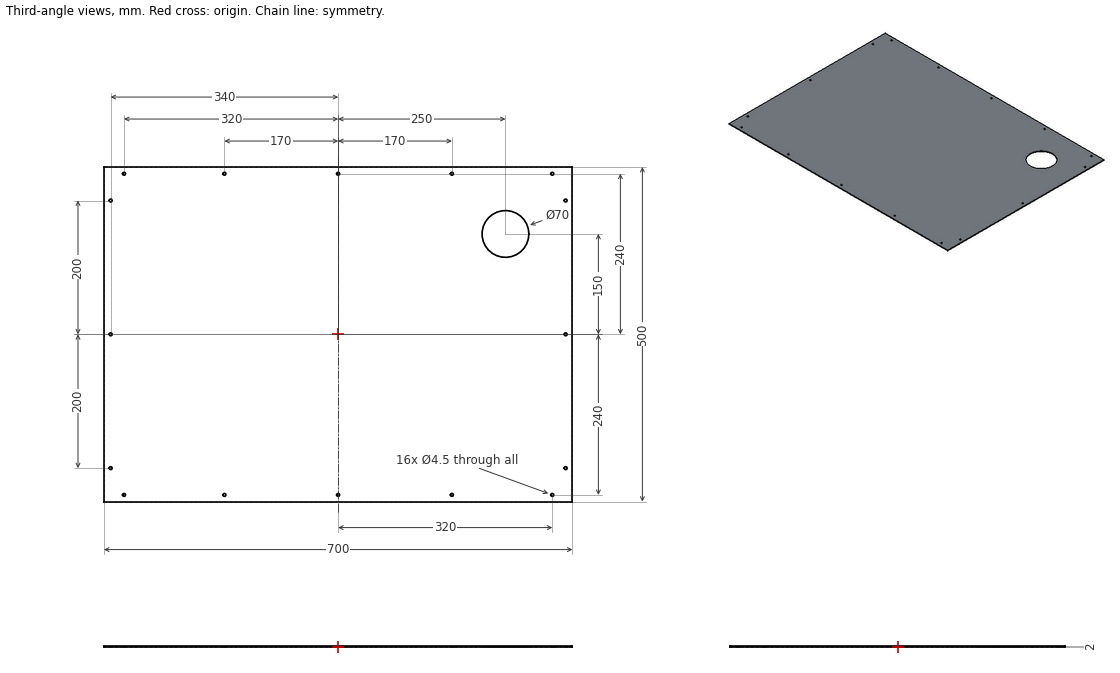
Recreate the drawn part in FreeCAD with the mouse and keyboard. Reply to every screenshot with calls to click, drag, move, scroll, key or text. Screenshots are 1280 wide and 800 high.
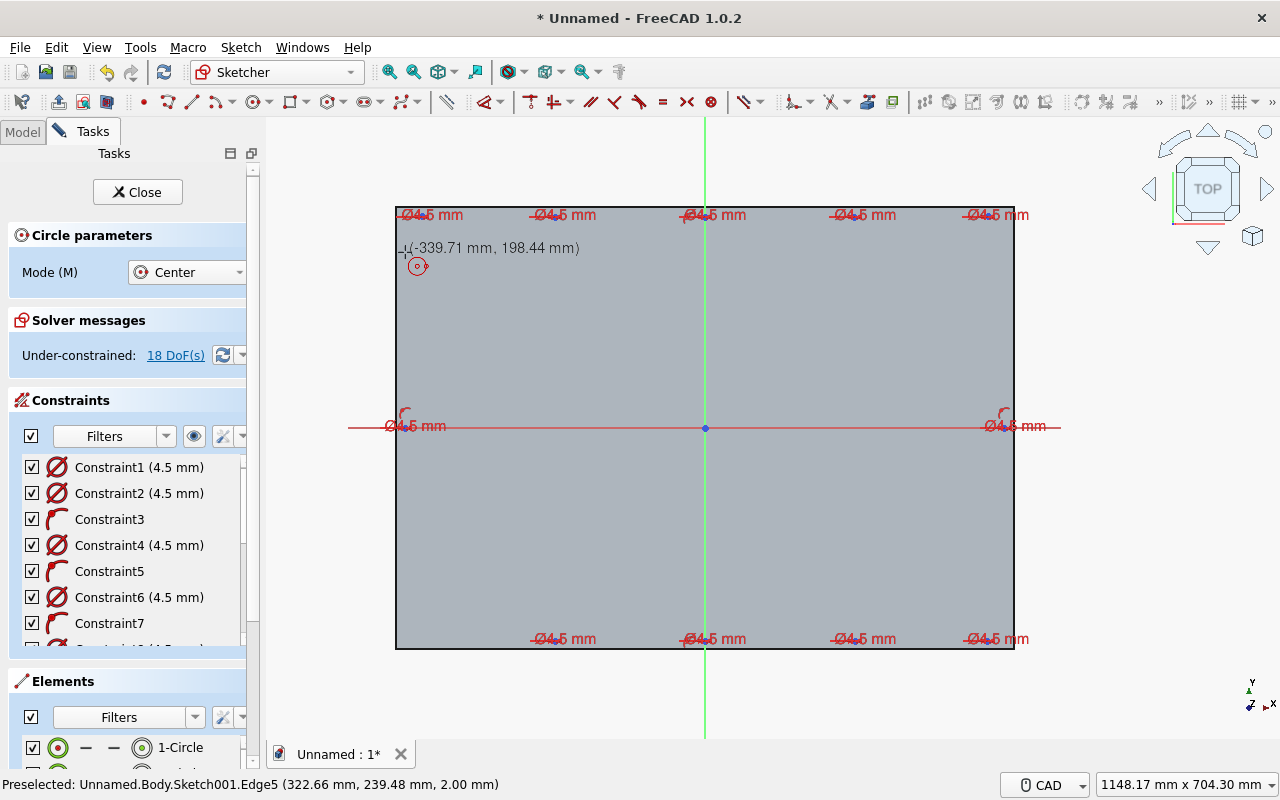
click(405, 252)
move(406, 250)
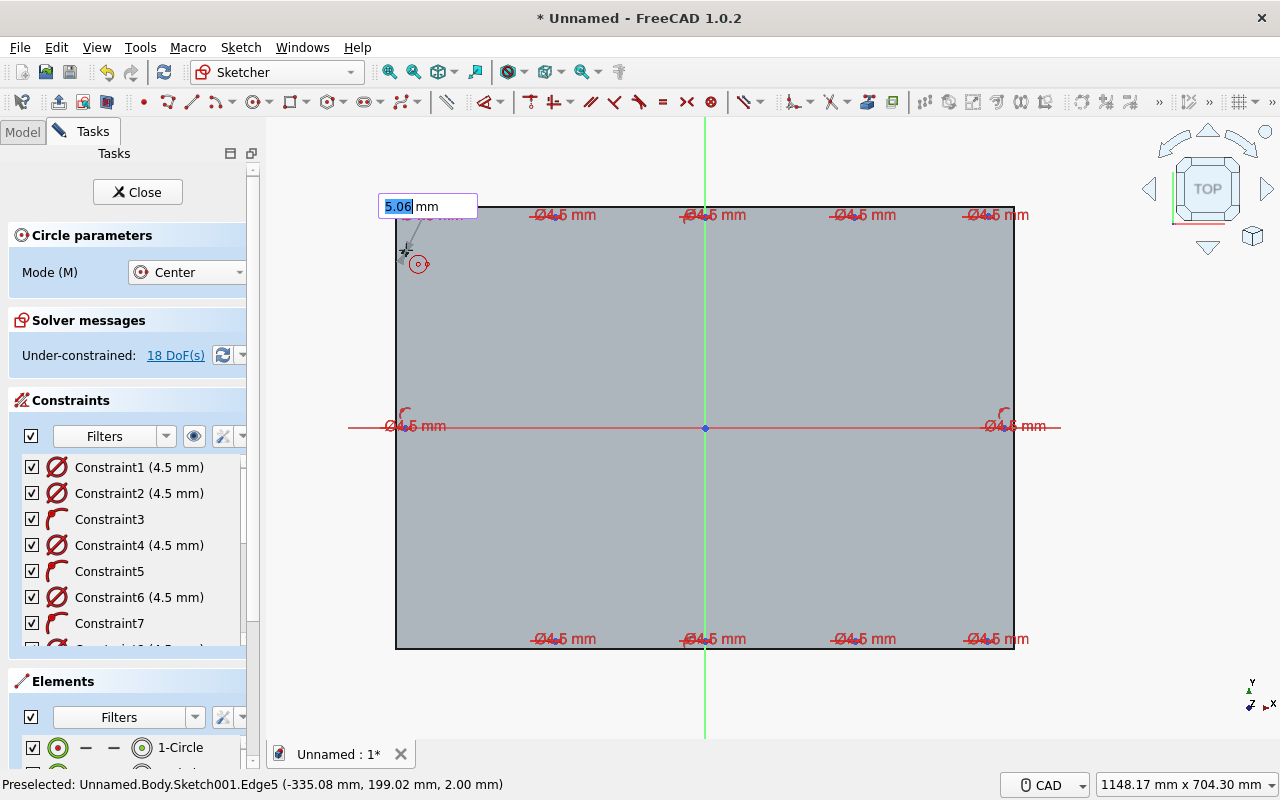
text(4.5)
key(Return)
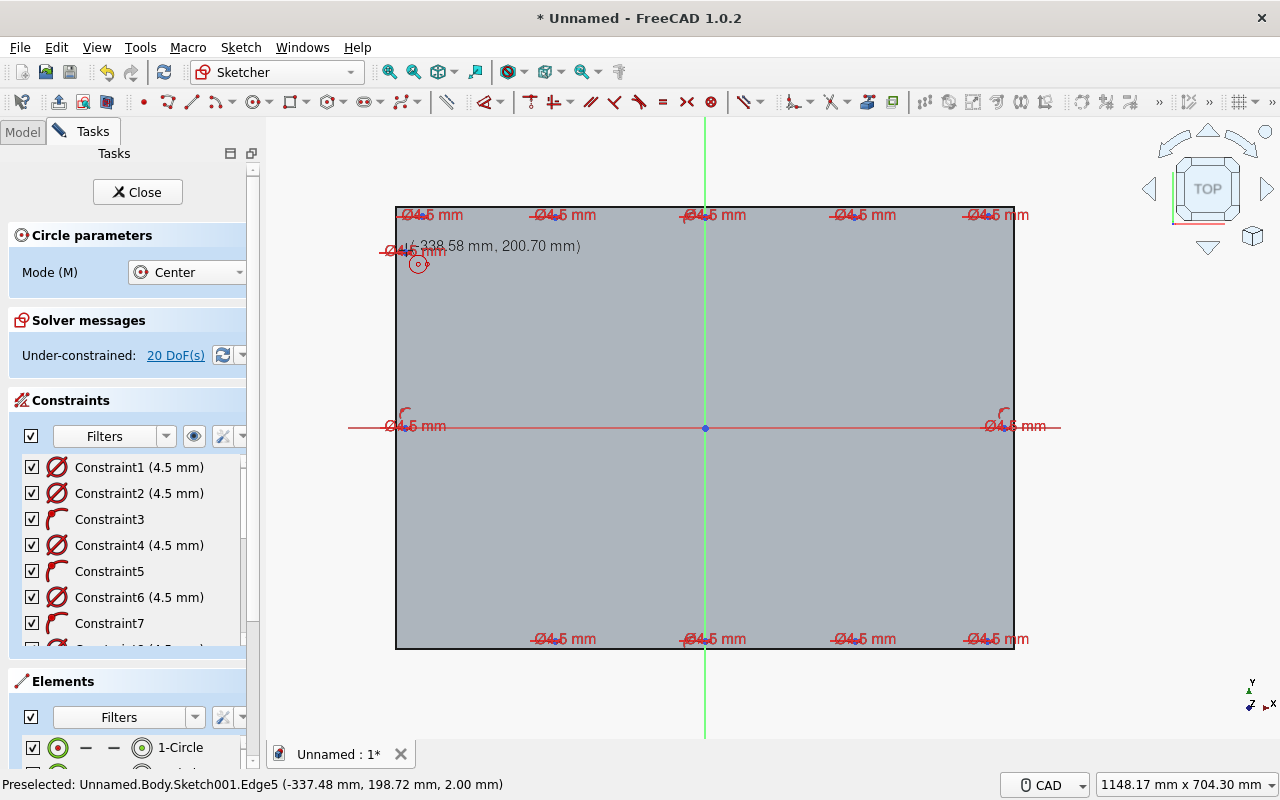
scroll(405, 605, up, 13)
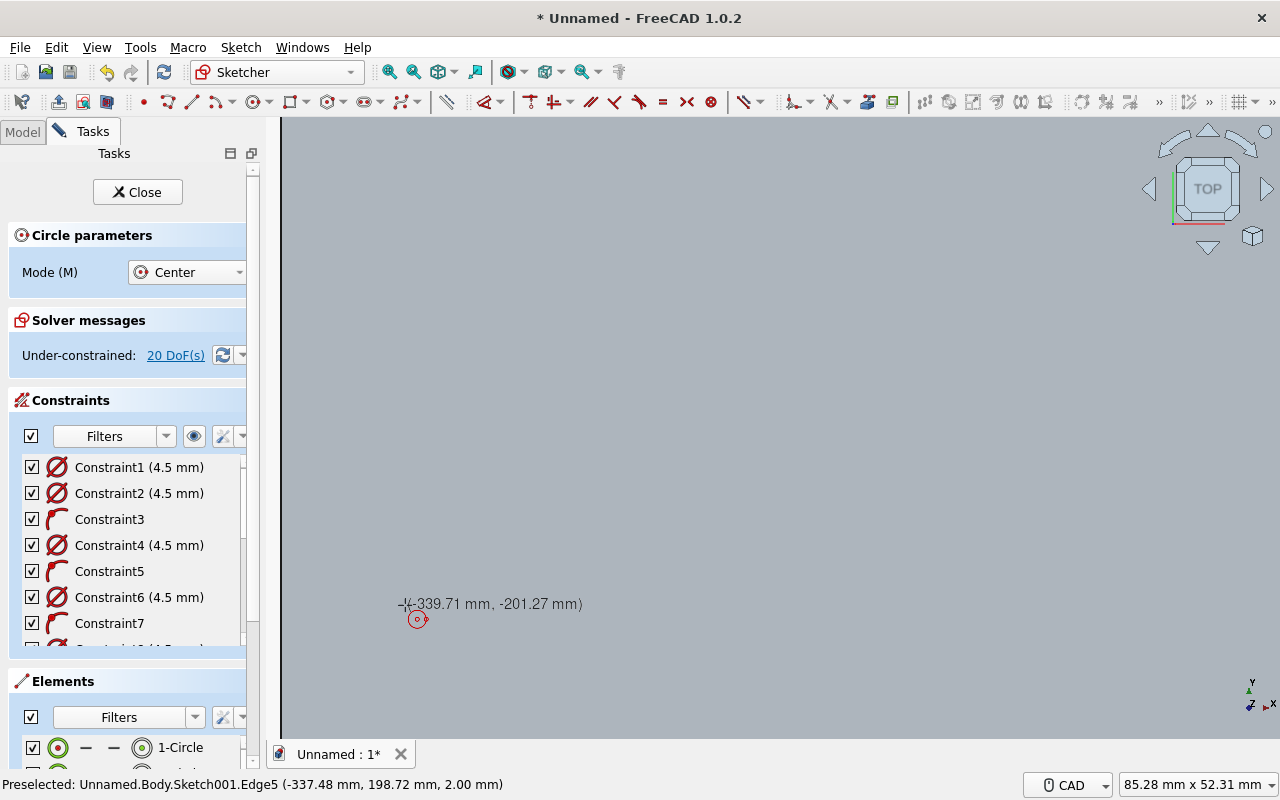
scroll(405, 606, down, 13)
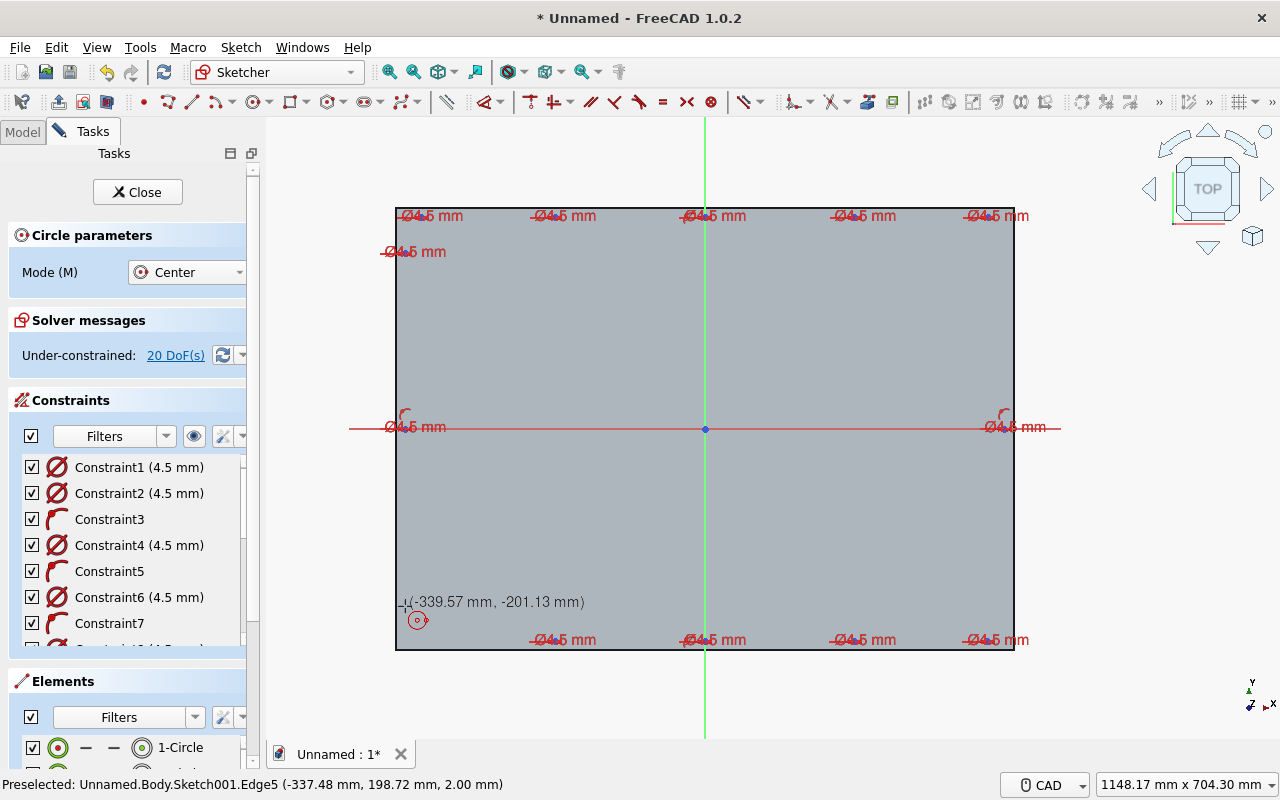
click(405, 606)
move(406, 604)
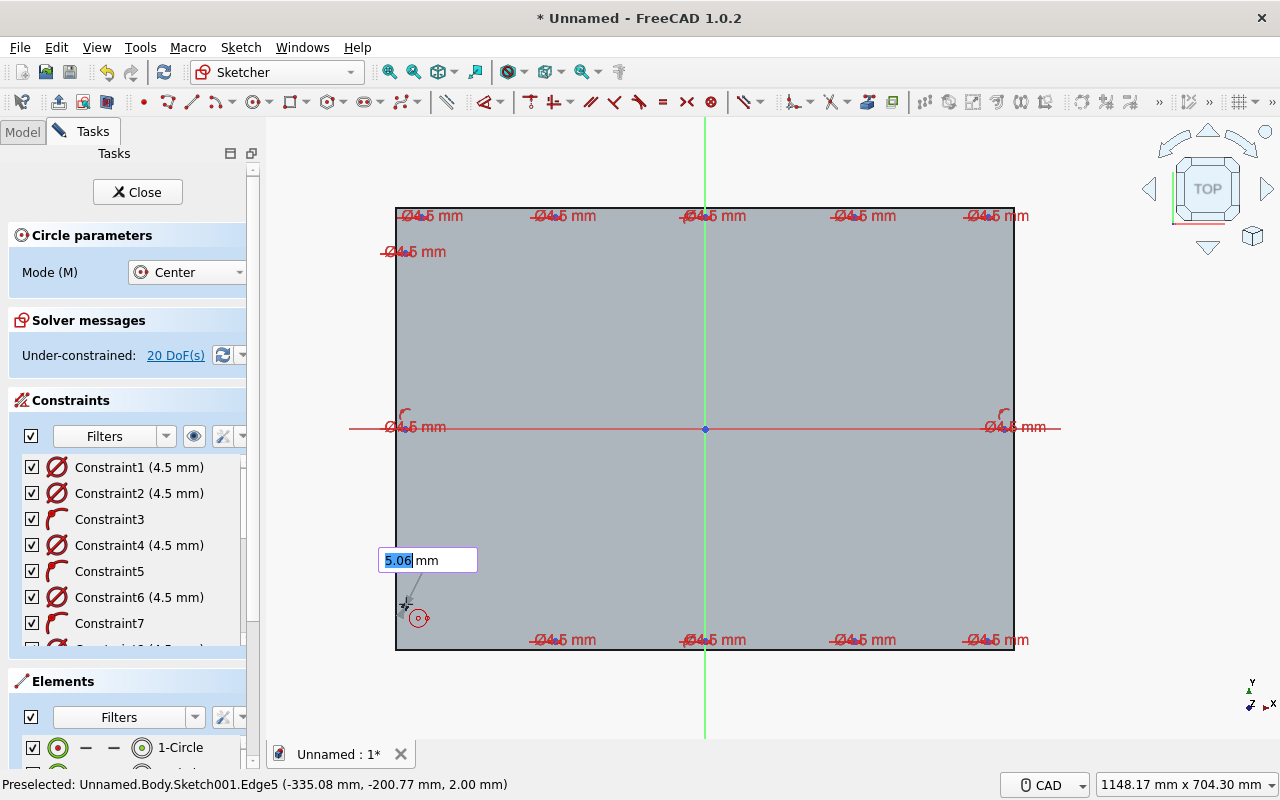
text(4.5)
key(Return)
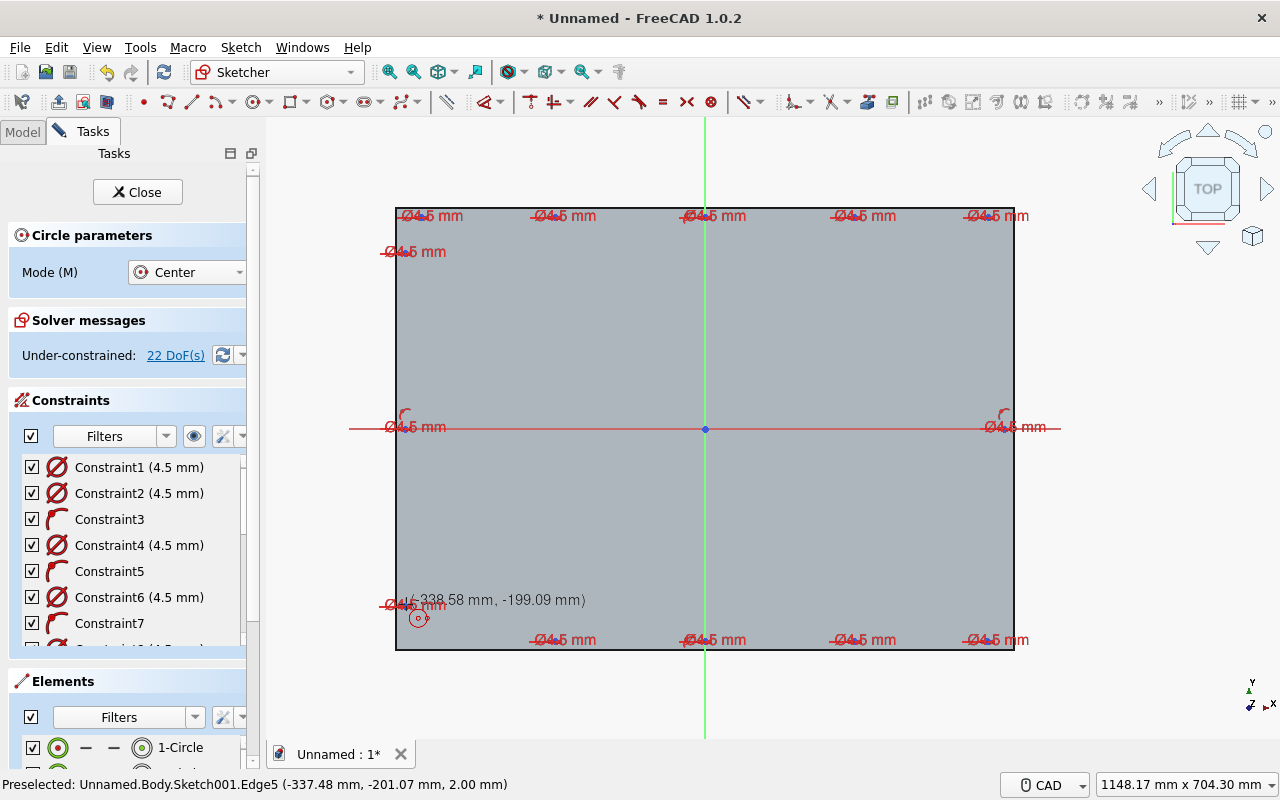
scroll(1005, 606, up, 13)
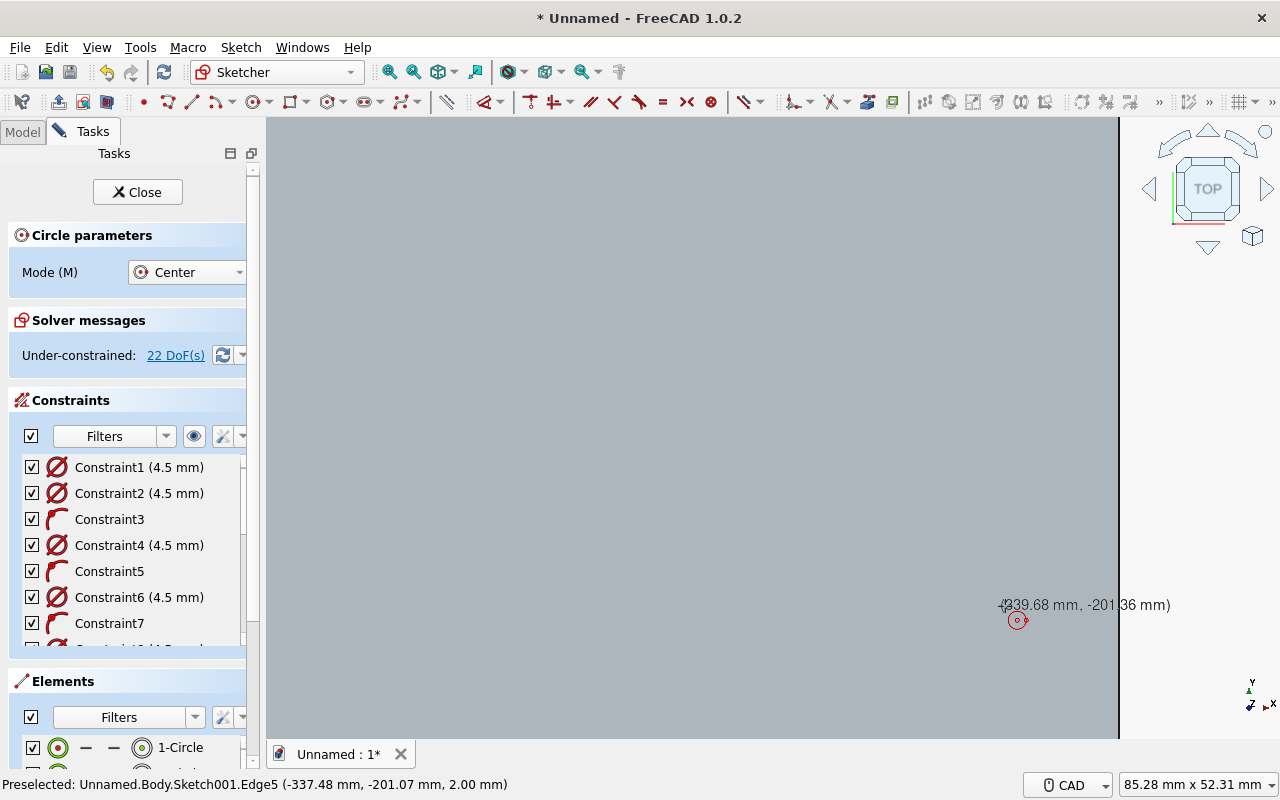
scroll(1005, 606, down, 13)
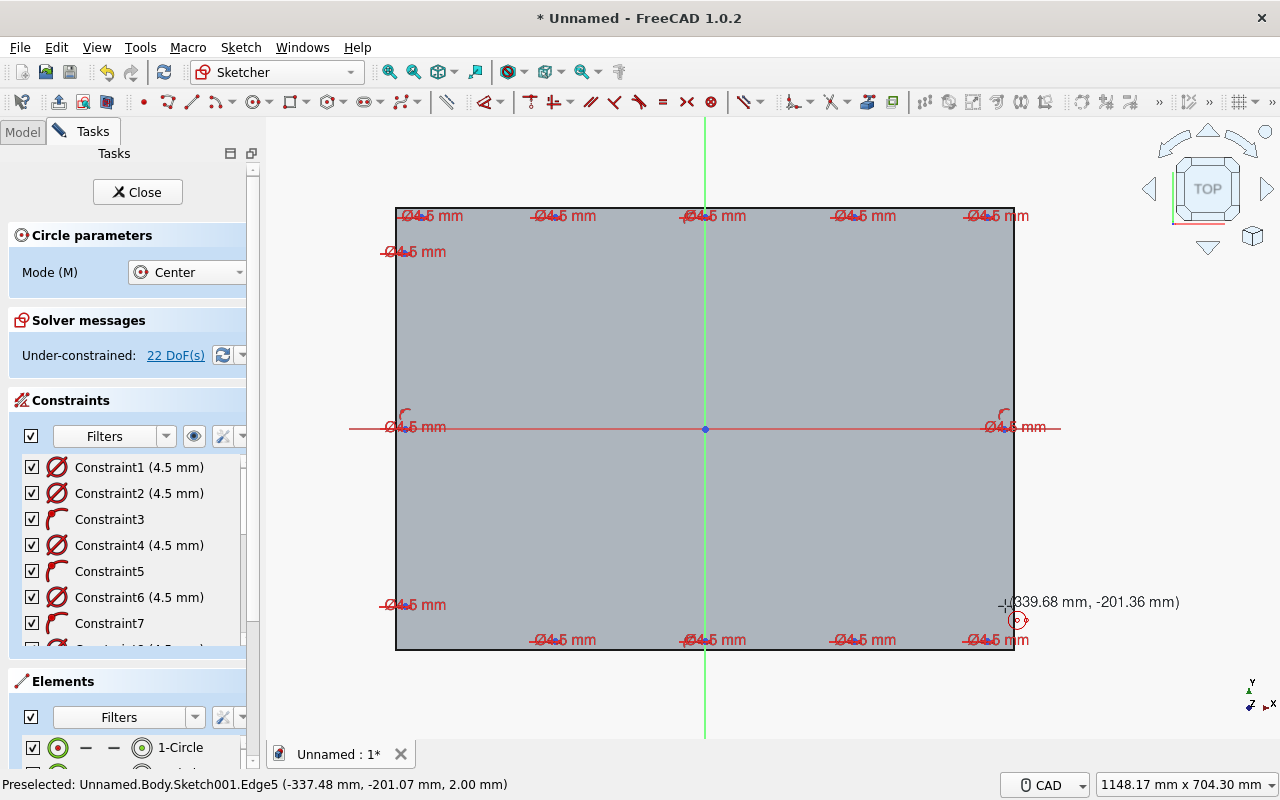
click(1005, 606)
move(1007, 604)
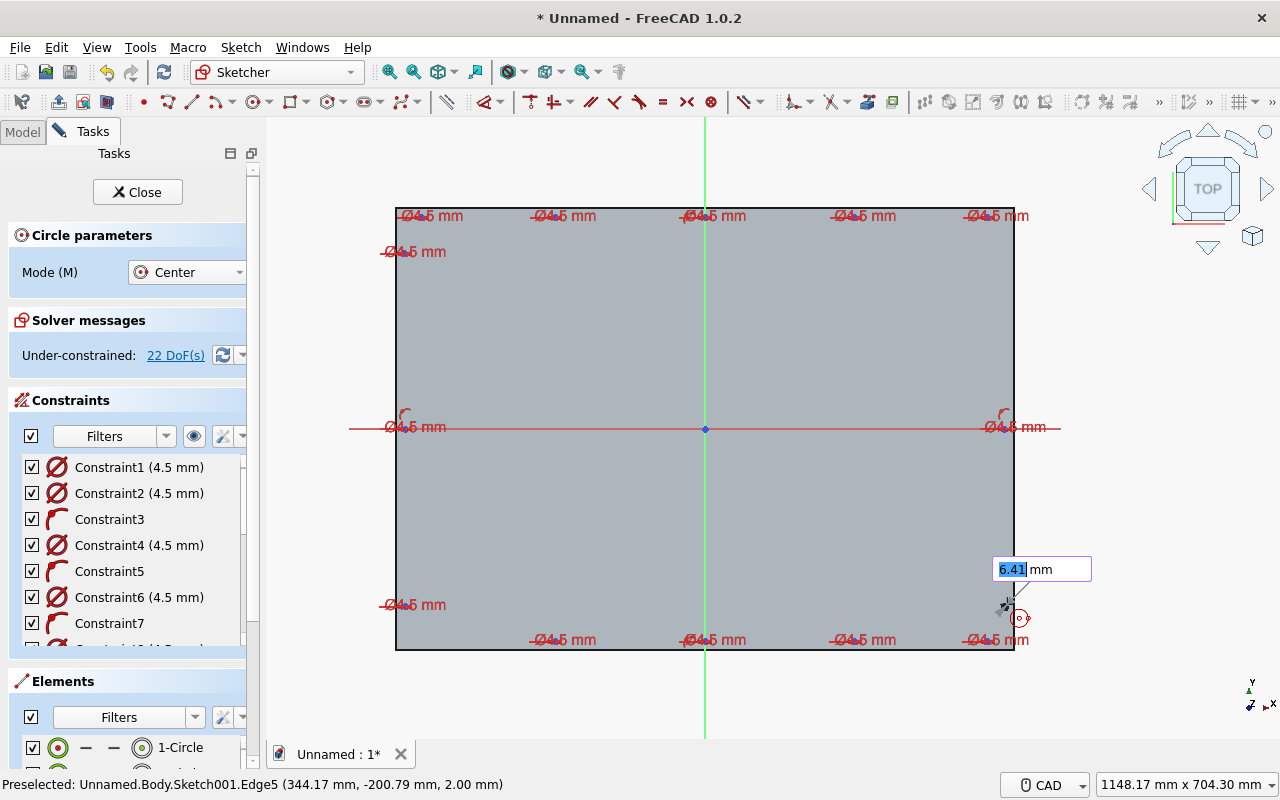
text(4.5)
key(Return)